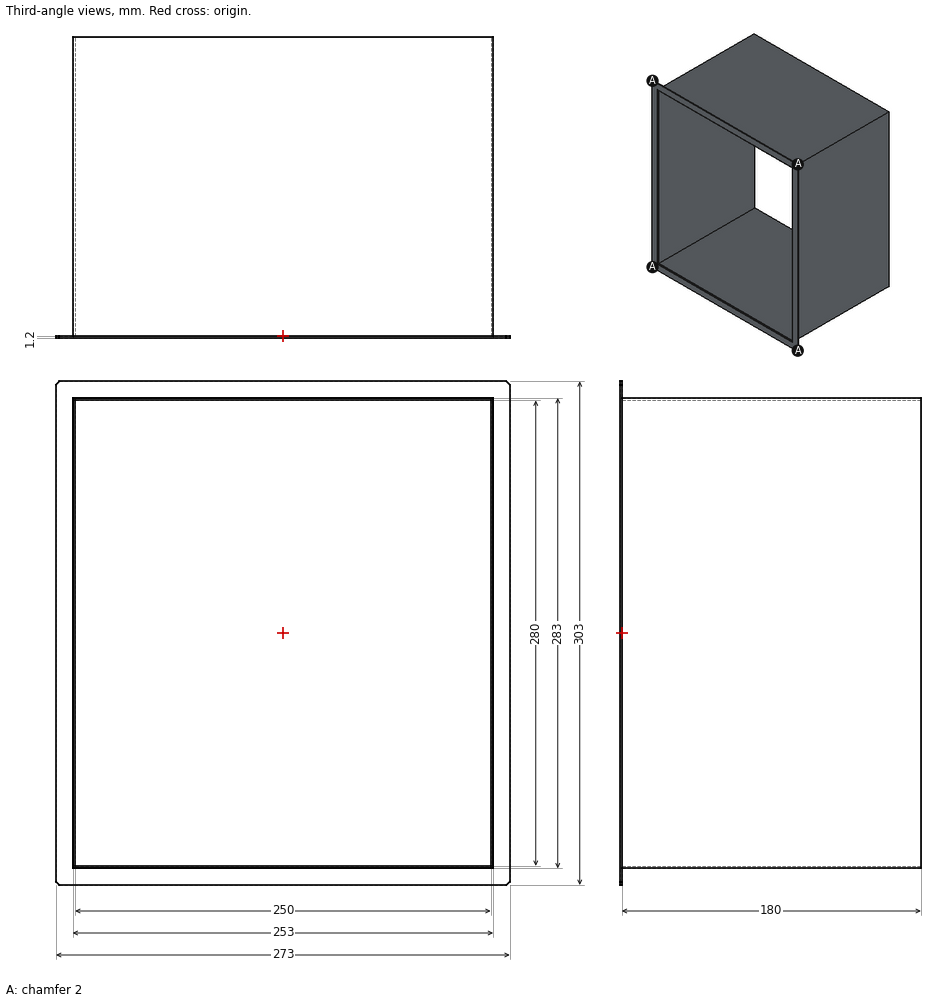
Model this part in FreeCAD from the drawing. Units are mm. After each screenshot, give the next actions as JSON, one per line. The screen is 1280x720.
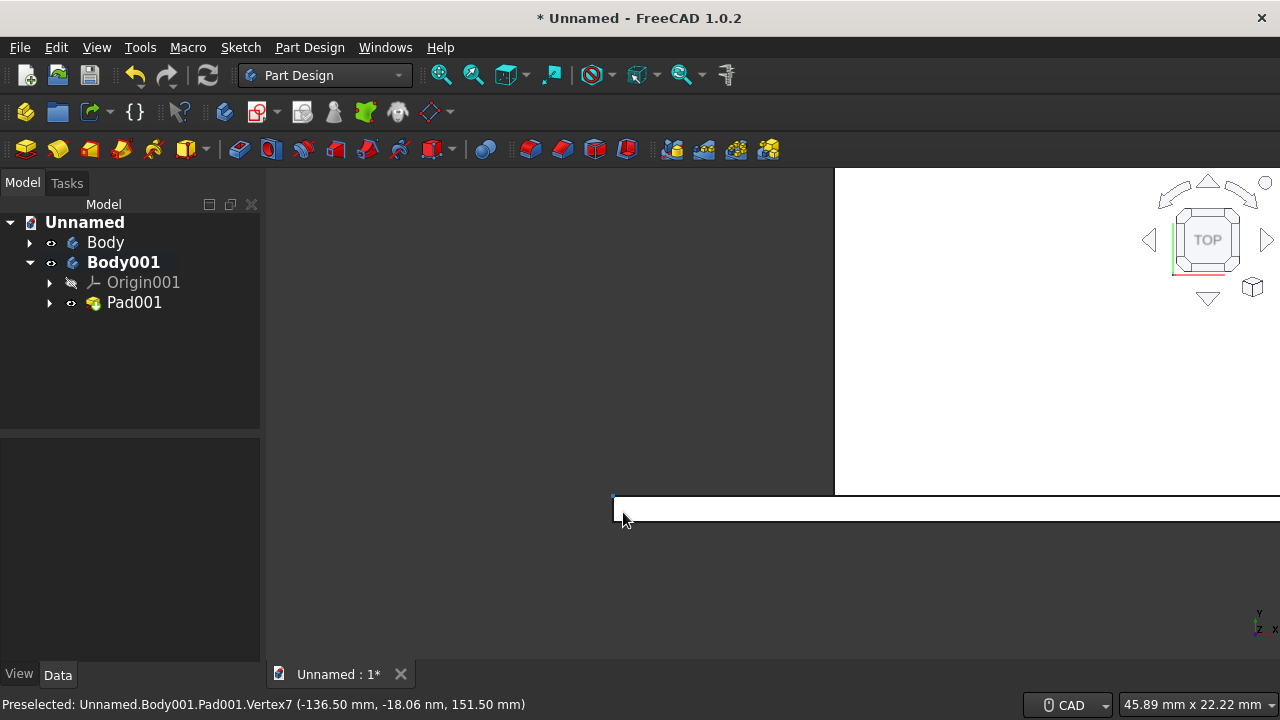
{"action": "left_click", "coordinate": [613, 508]}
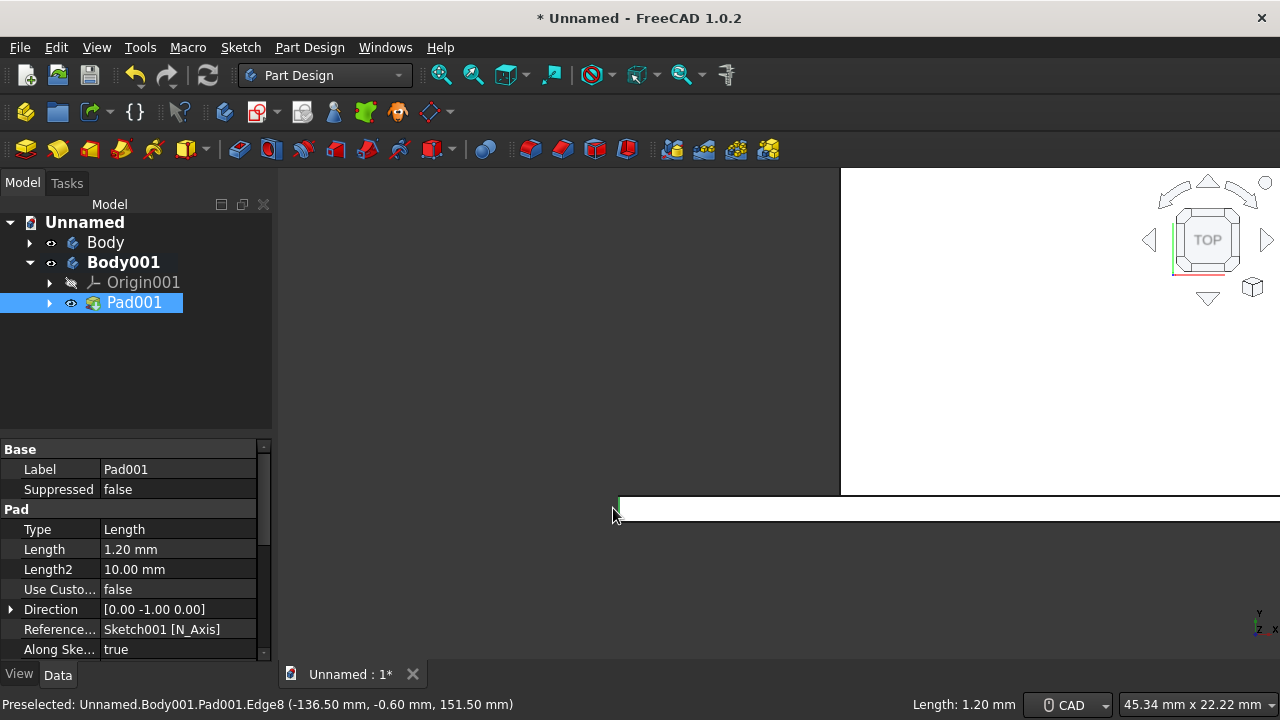
{"action": "key", "text": "v f"}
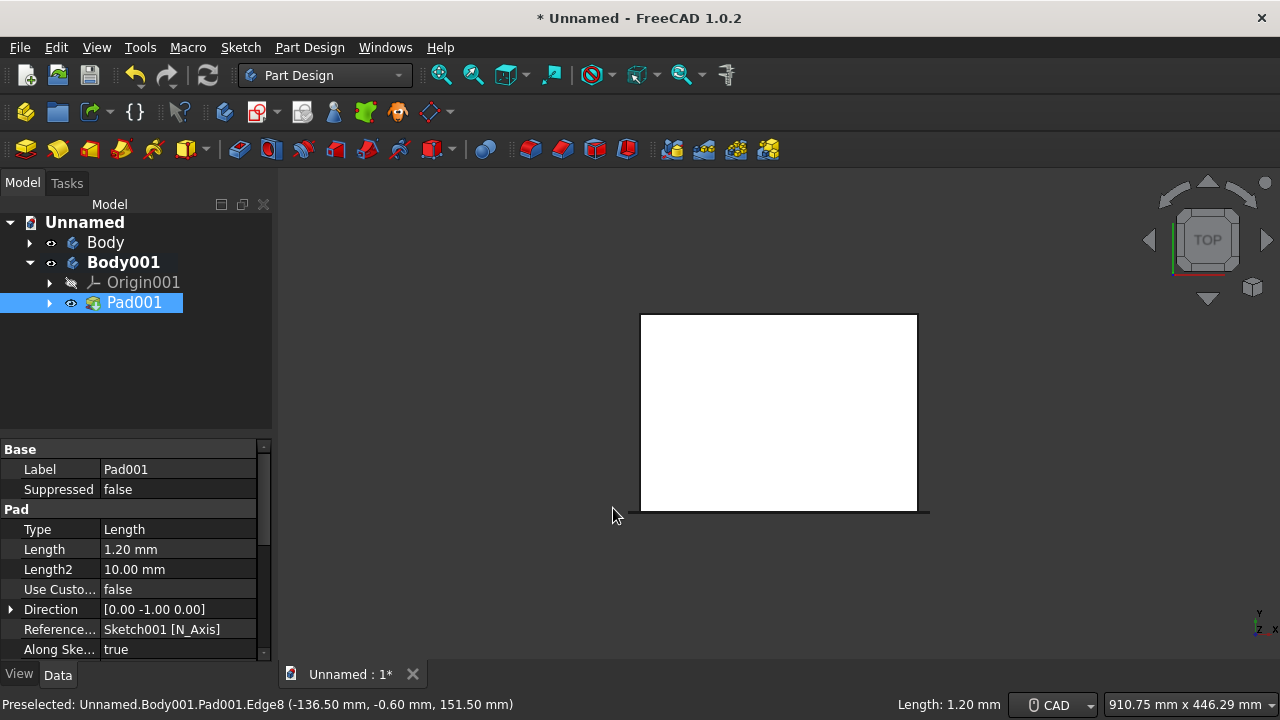
{"action": "key", "text": "1"}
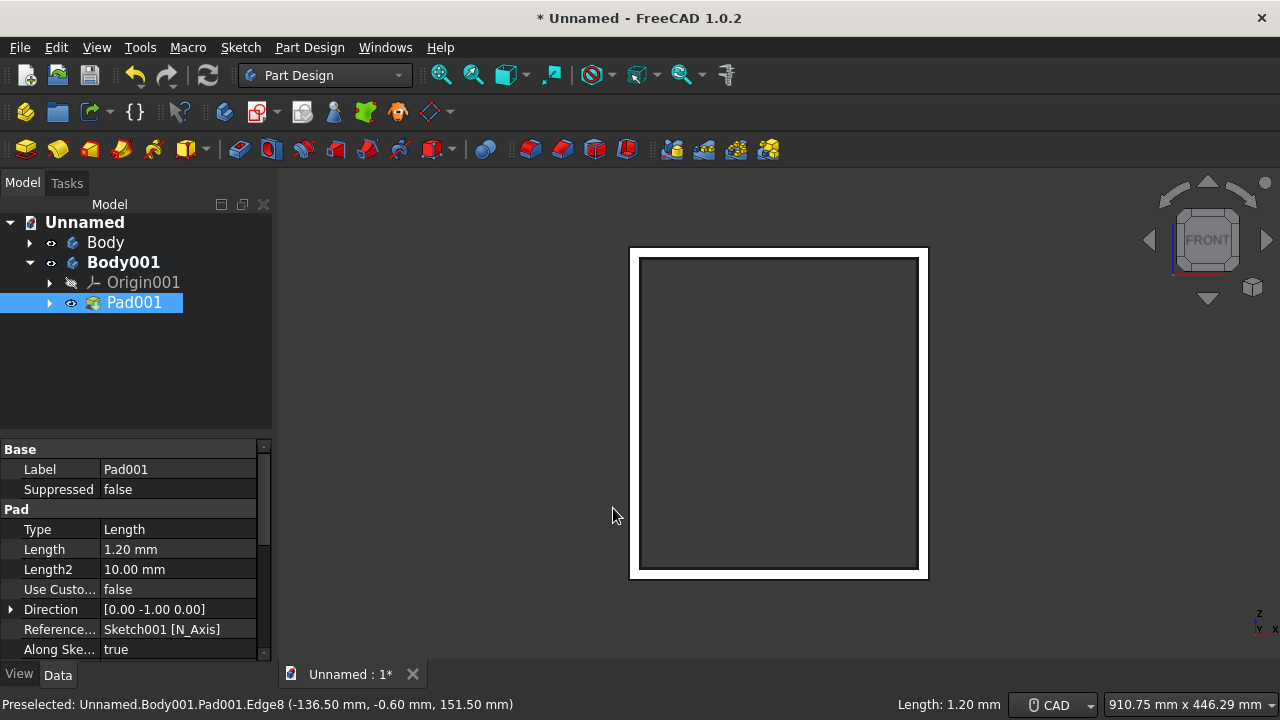
{"action": "scroll", "coordinate": [629, 579], "scroll_direction": "up", "scroll_amount": 15}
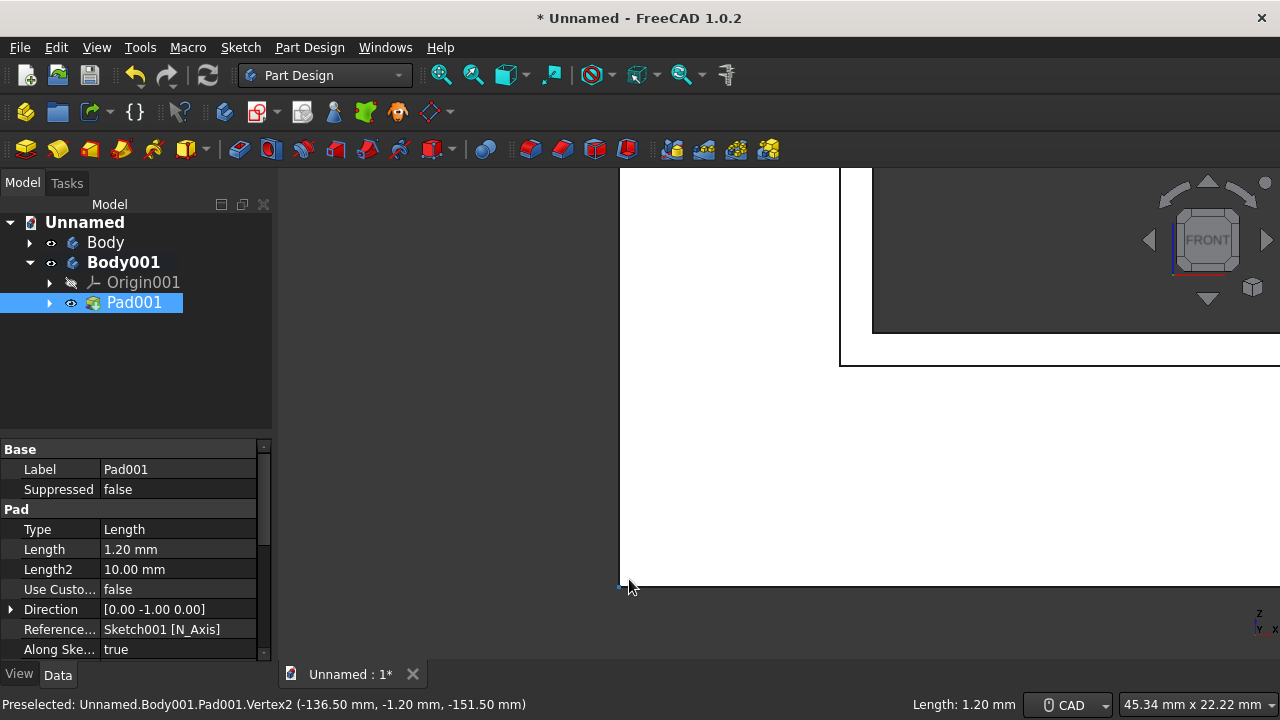
{"action": "left_click", "coordinate": [442, 76]}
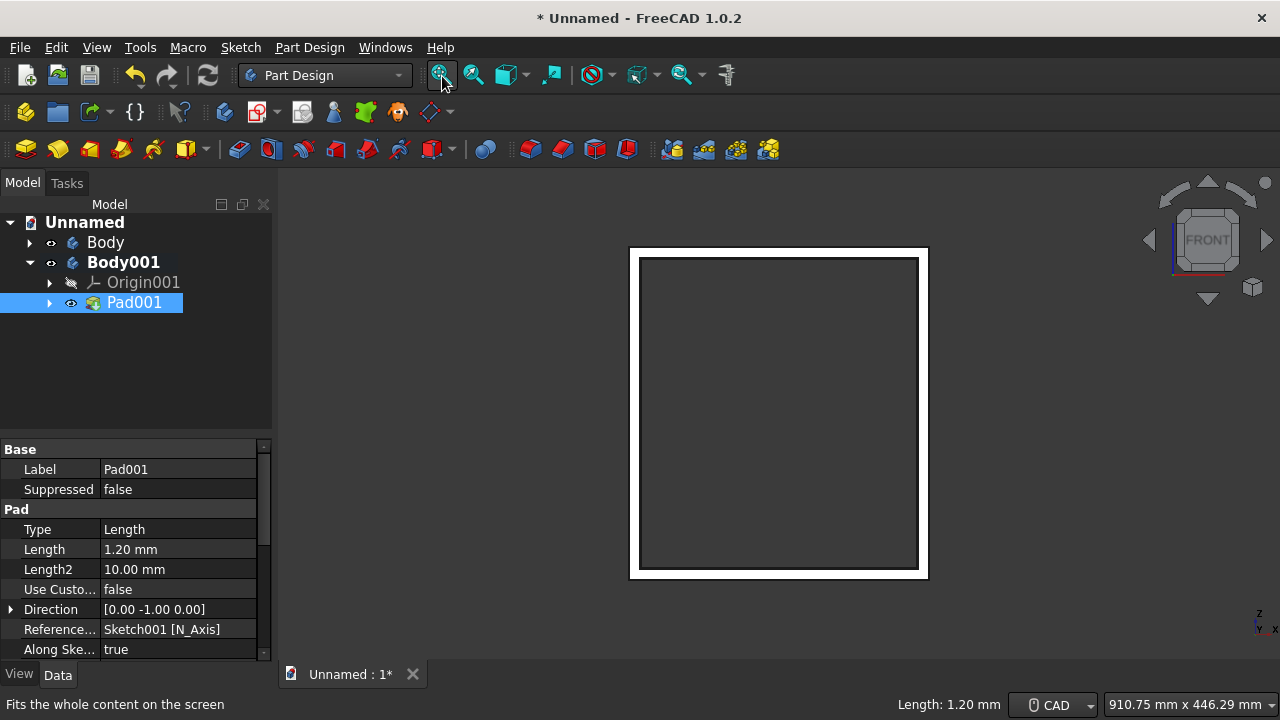
{"action": "key", "text": "3"}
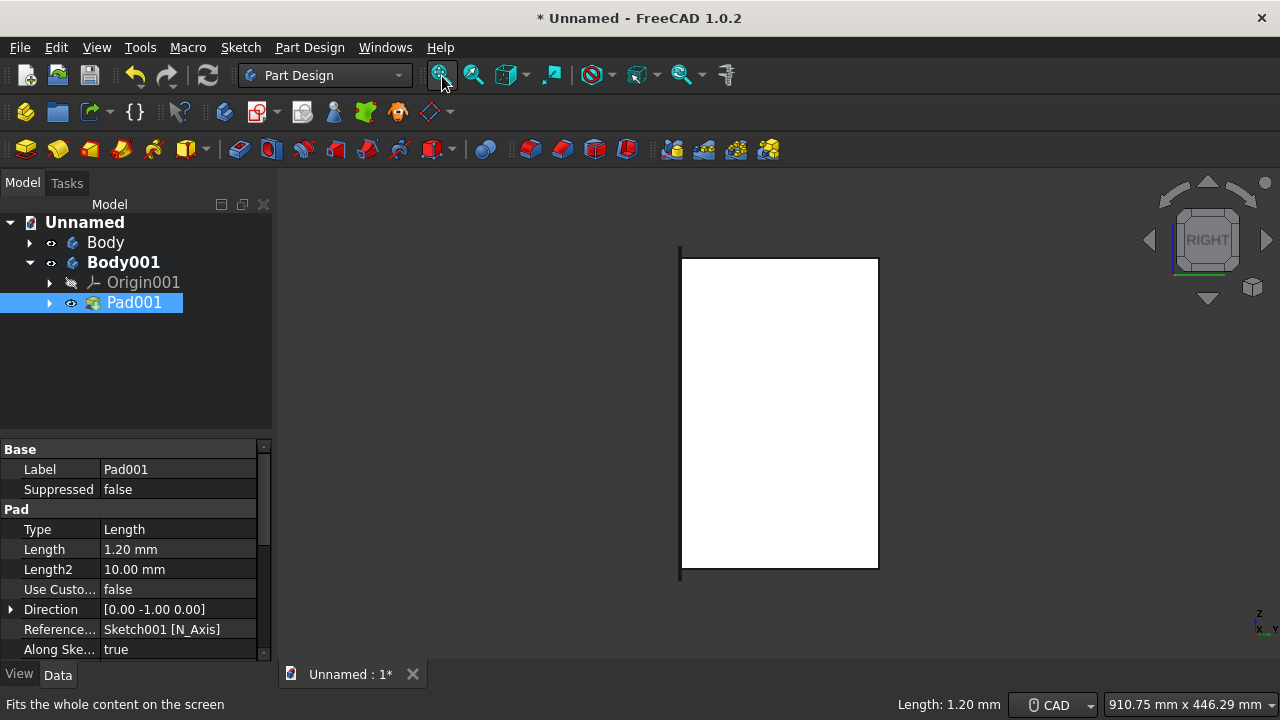
{"action": "scroll", "coordinate": [680, 579], "scroll_direction": "up", "scroll_amount": 15}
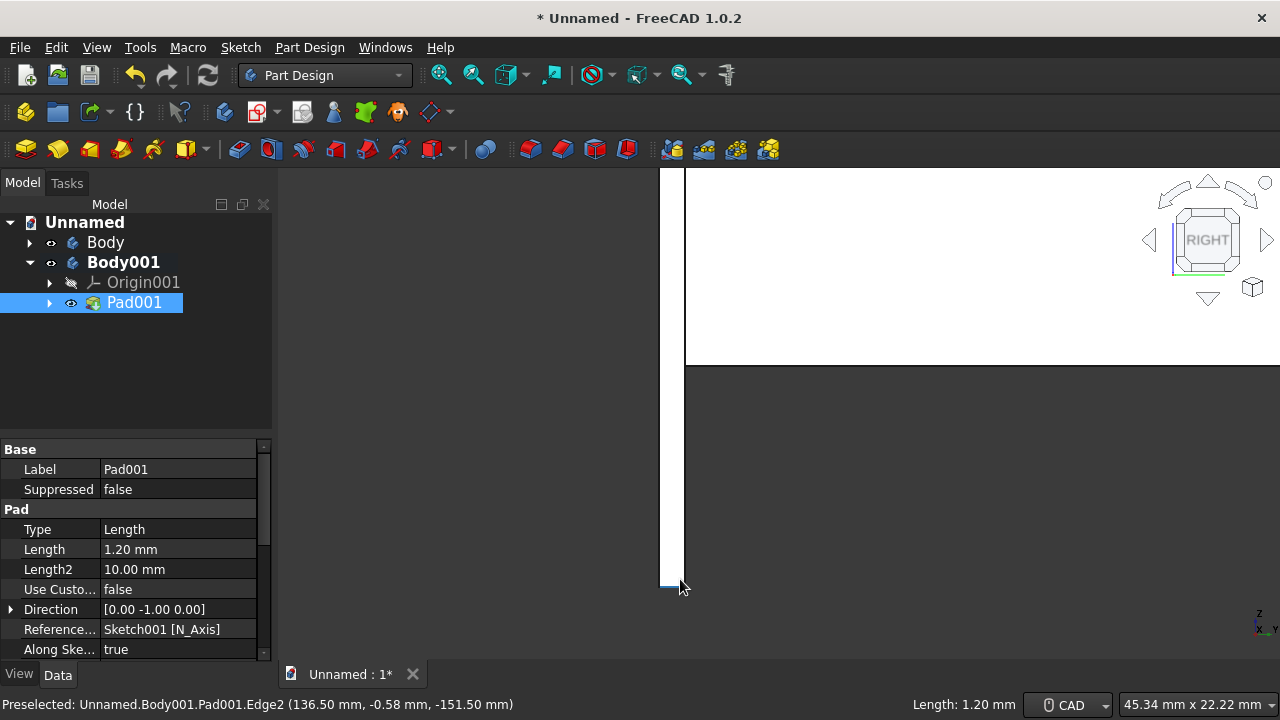
{"action": "left_click", "coordinate": [672, 586], "text": "ctrl"}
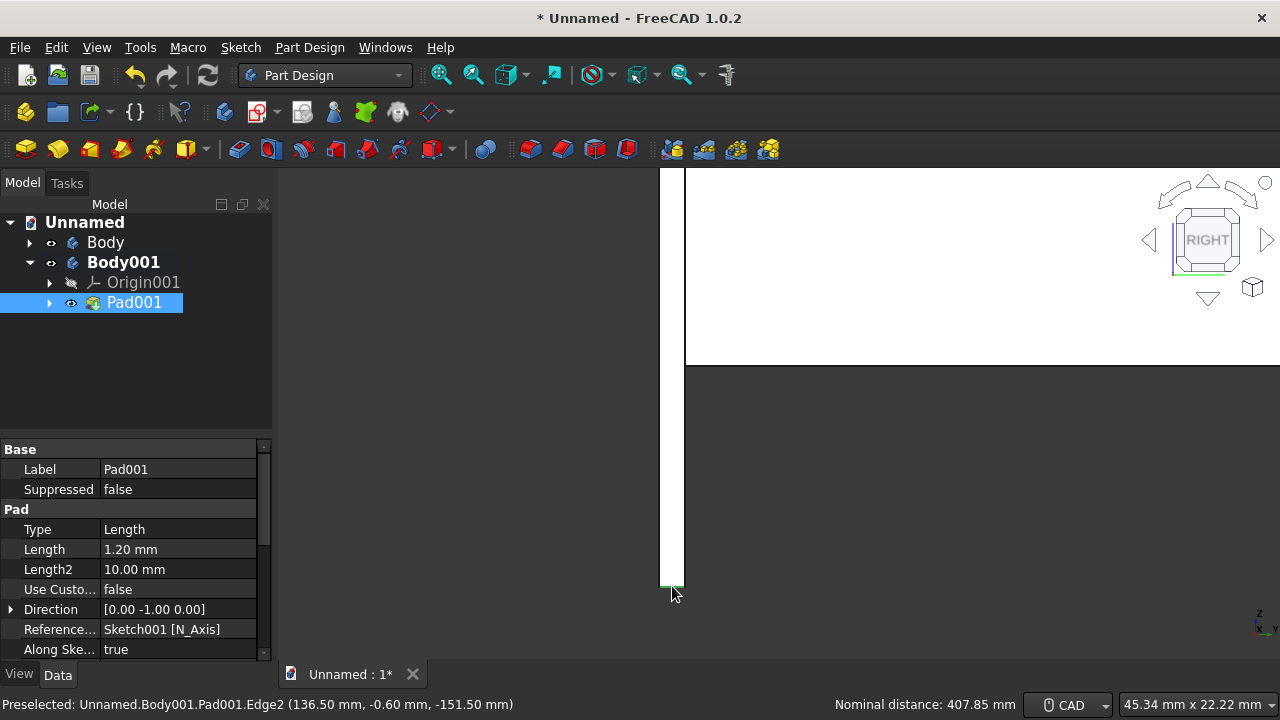
{"action": "left_click", "coordinate": [442, 76]}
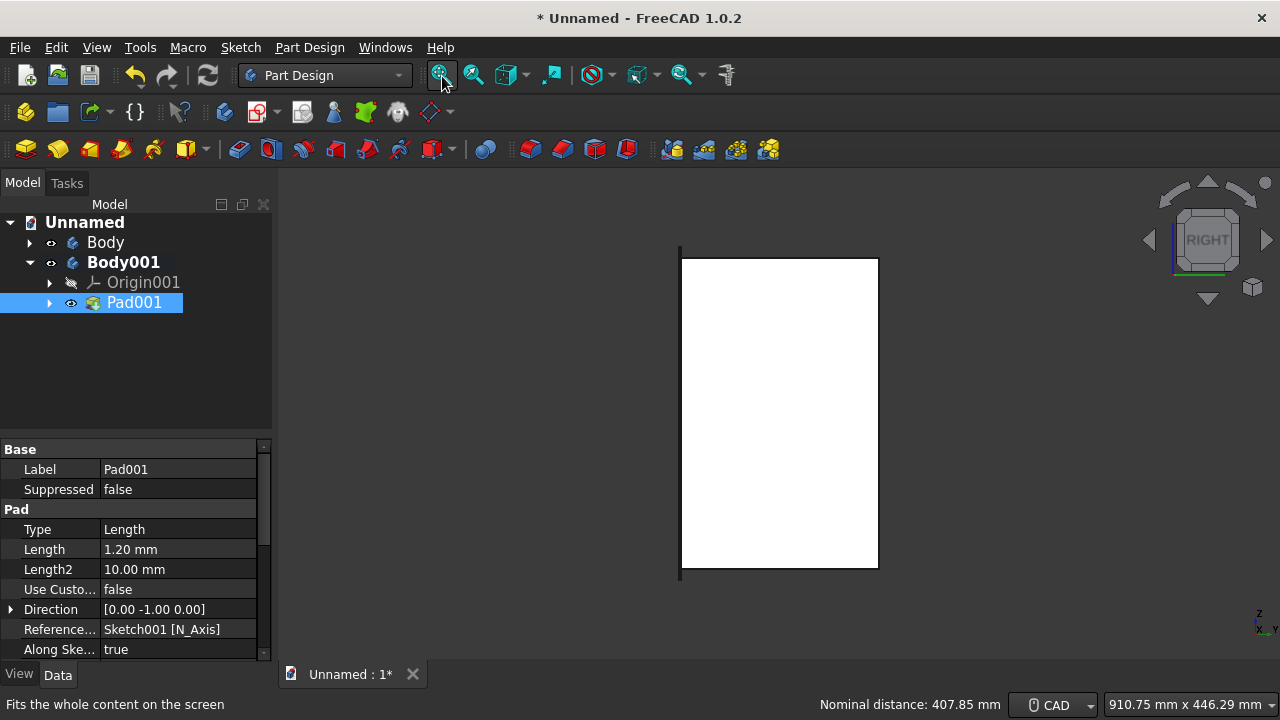
{"action": "key", "text": "5"}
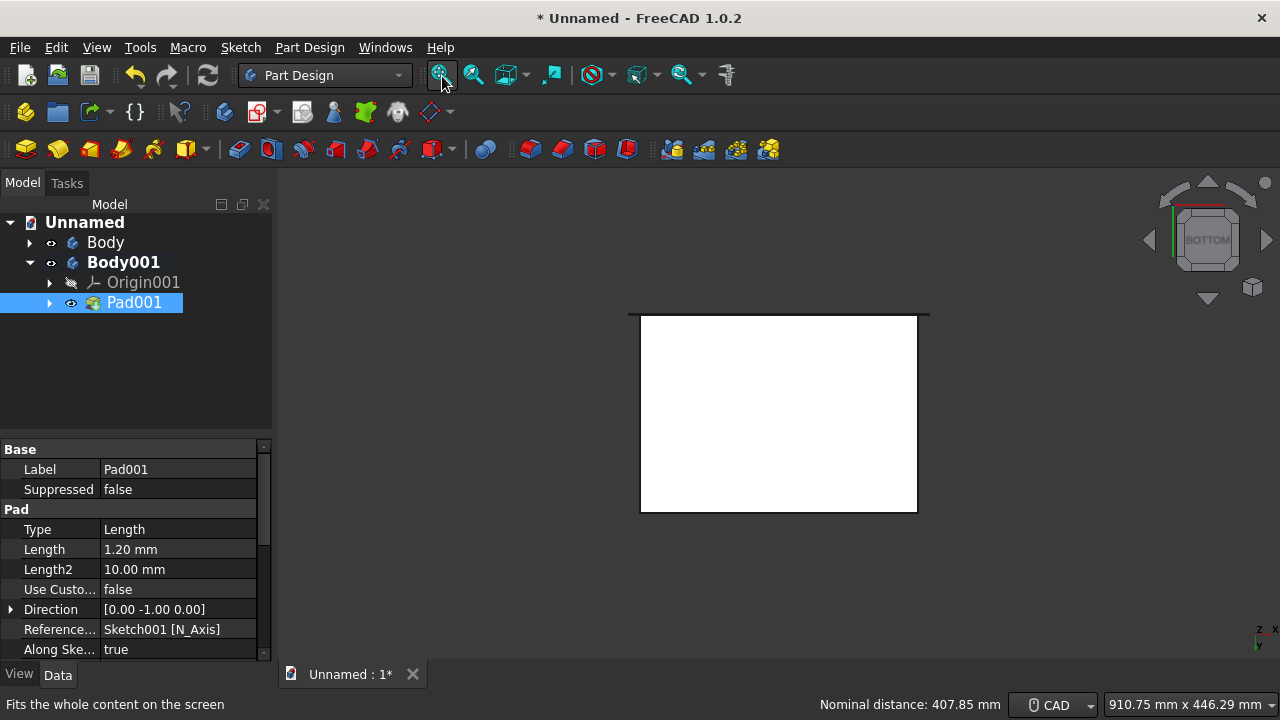
{"action": "left_click", "coordinate": [442, 76]}